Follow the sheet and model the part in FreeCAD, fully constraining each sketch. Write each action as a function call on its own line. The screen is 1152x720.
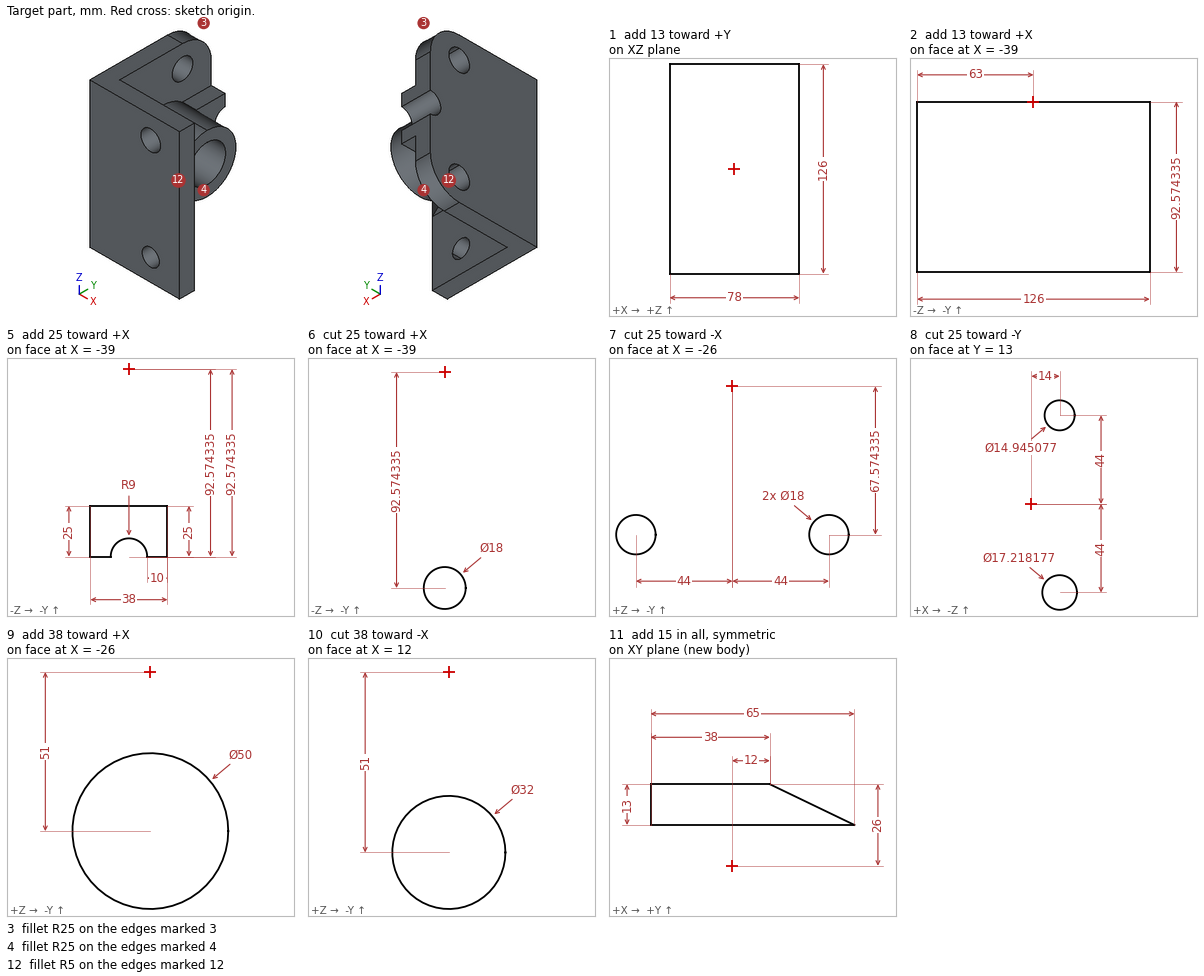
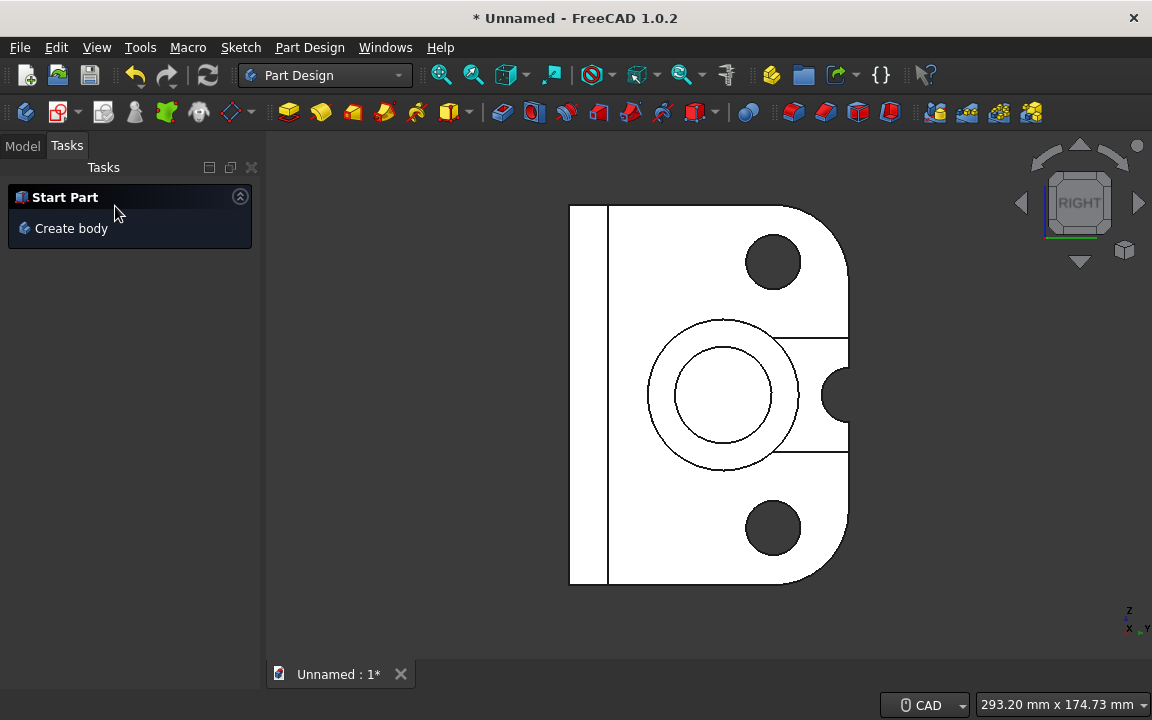
click(26, 112)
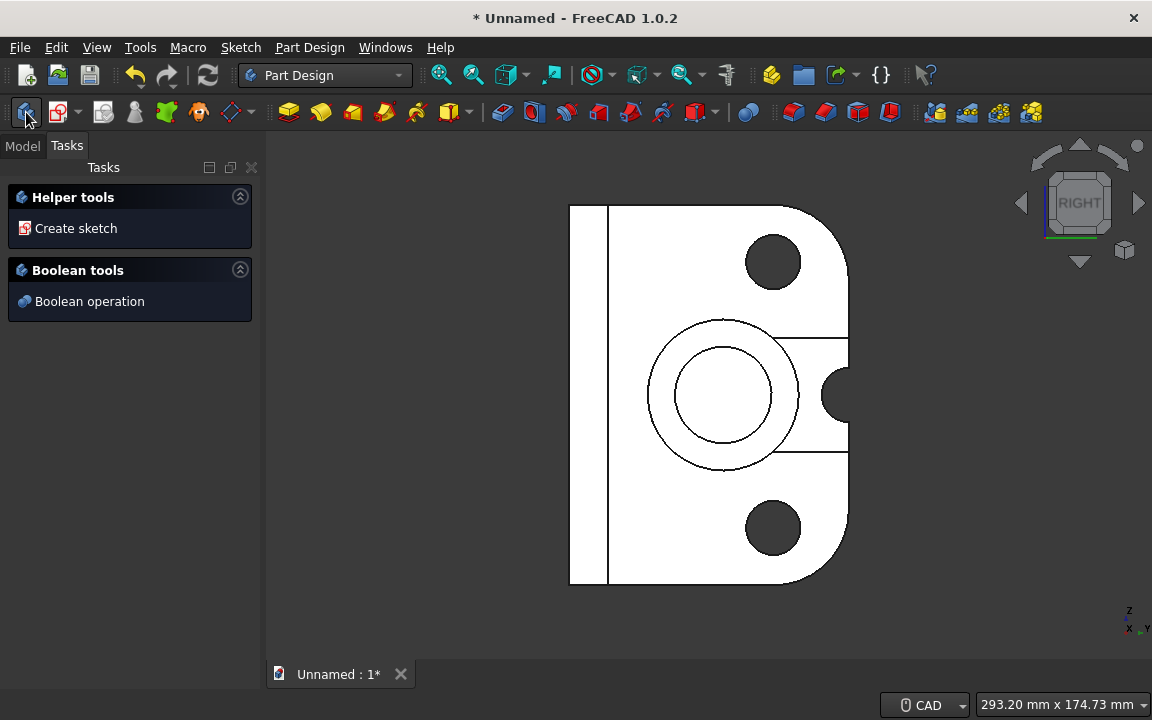
click(306, 619)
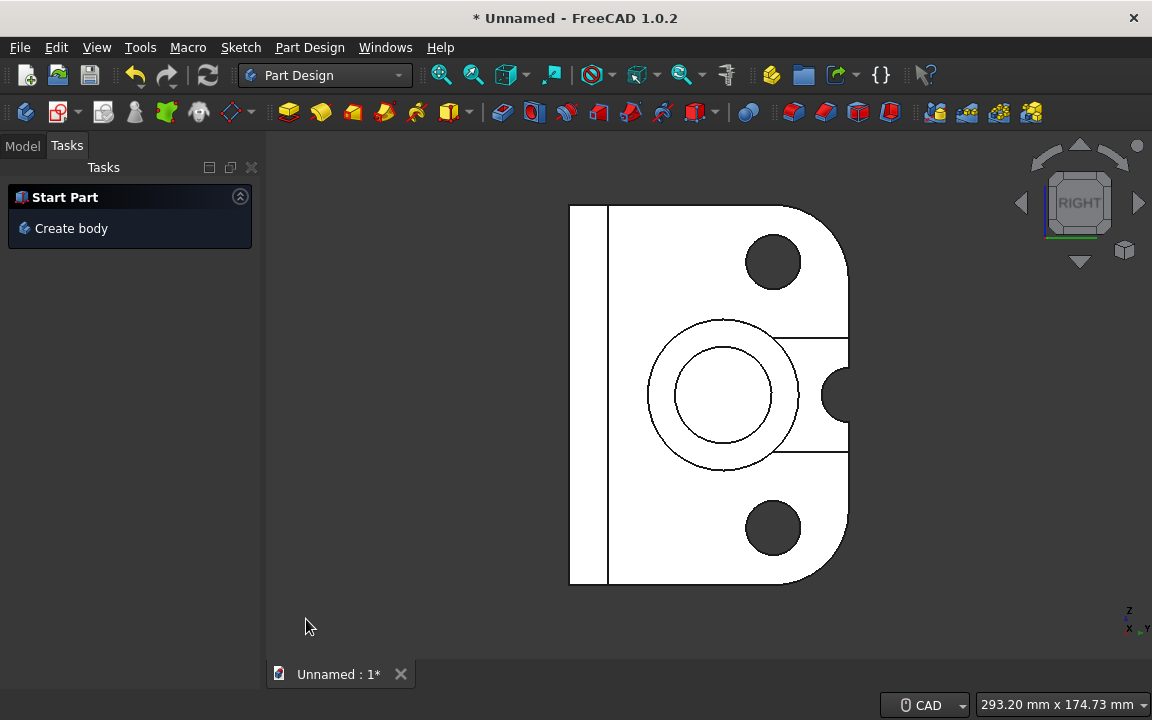
click(58, 112)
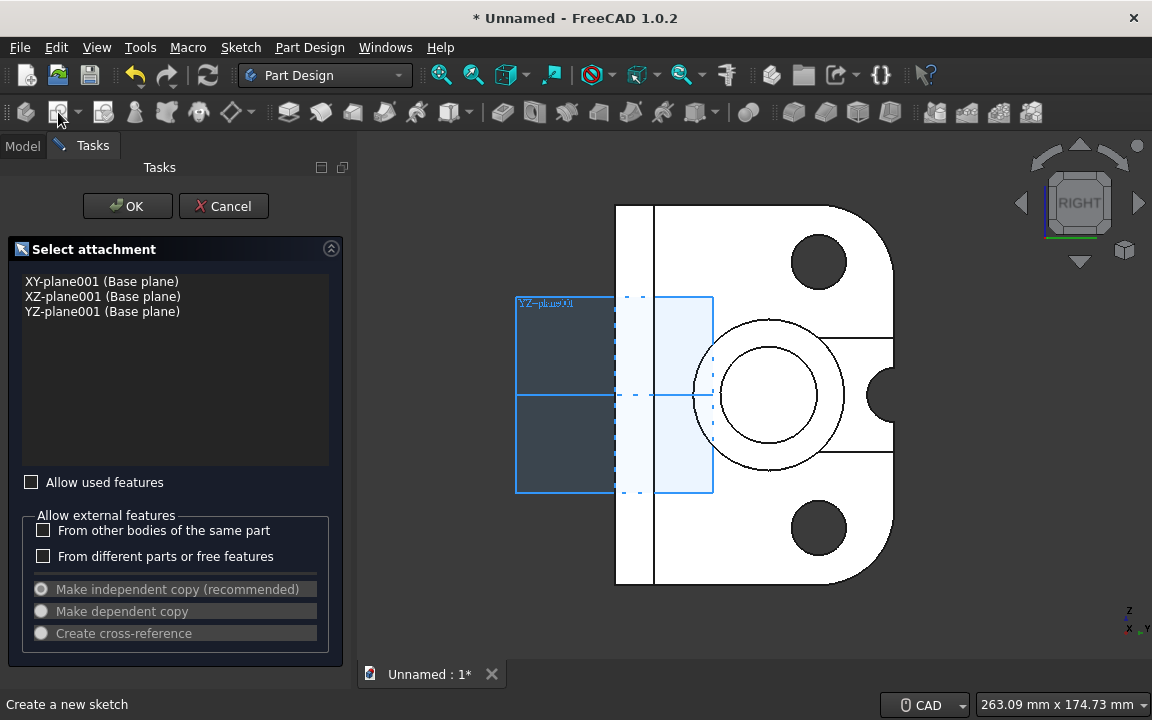
click(82, 282)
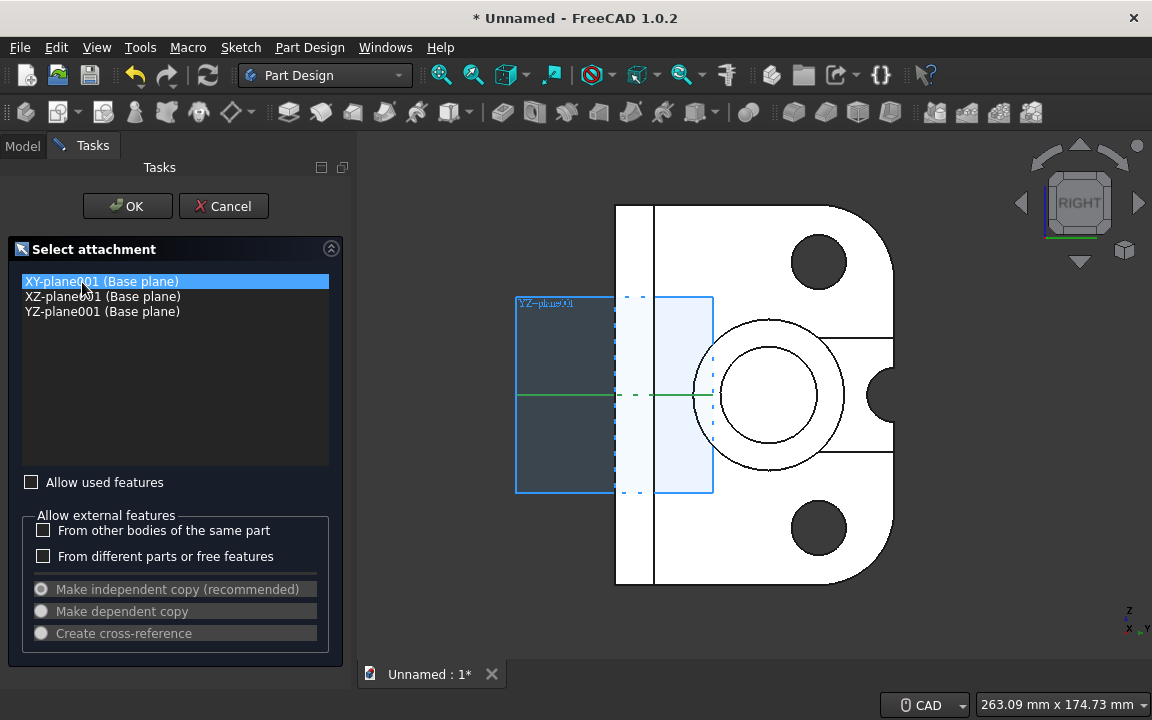
click(128, 206)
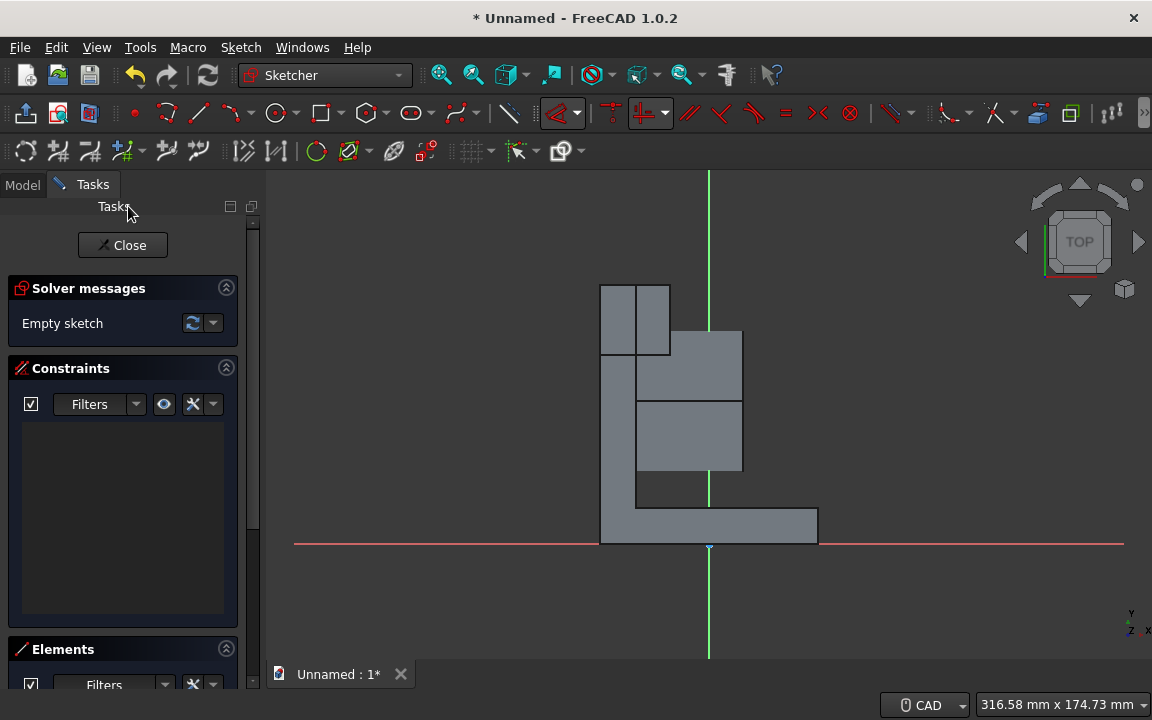
scroll(778, 562, up, 5)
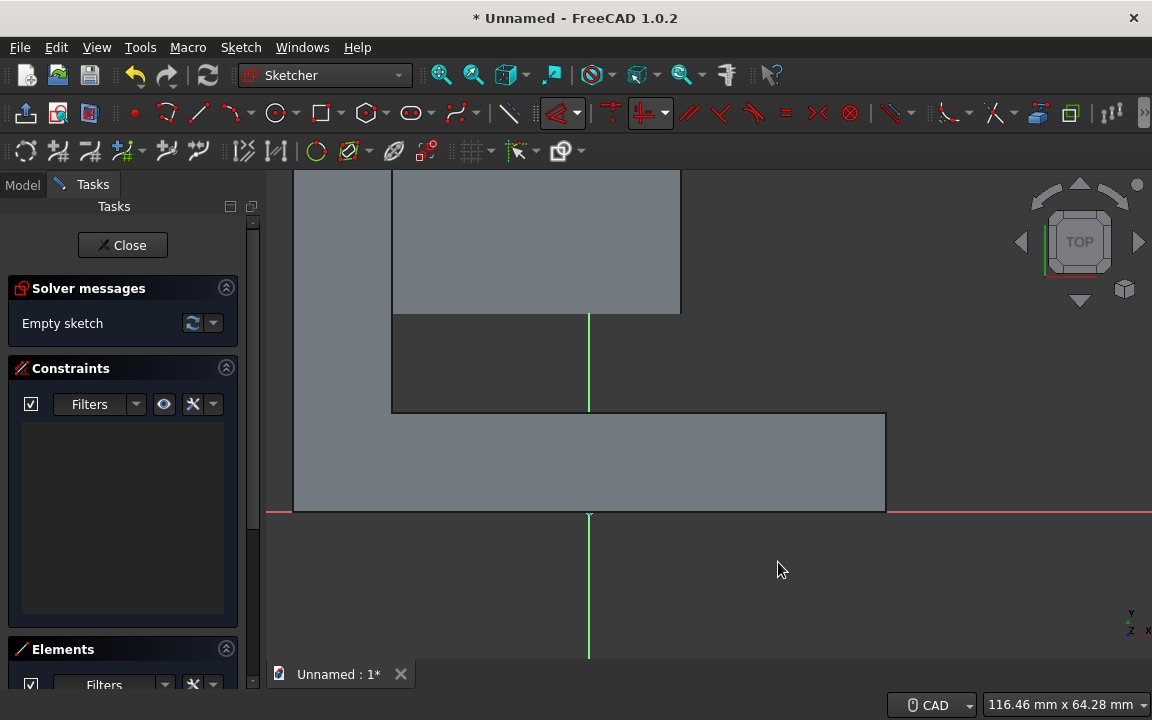
click(168, 114)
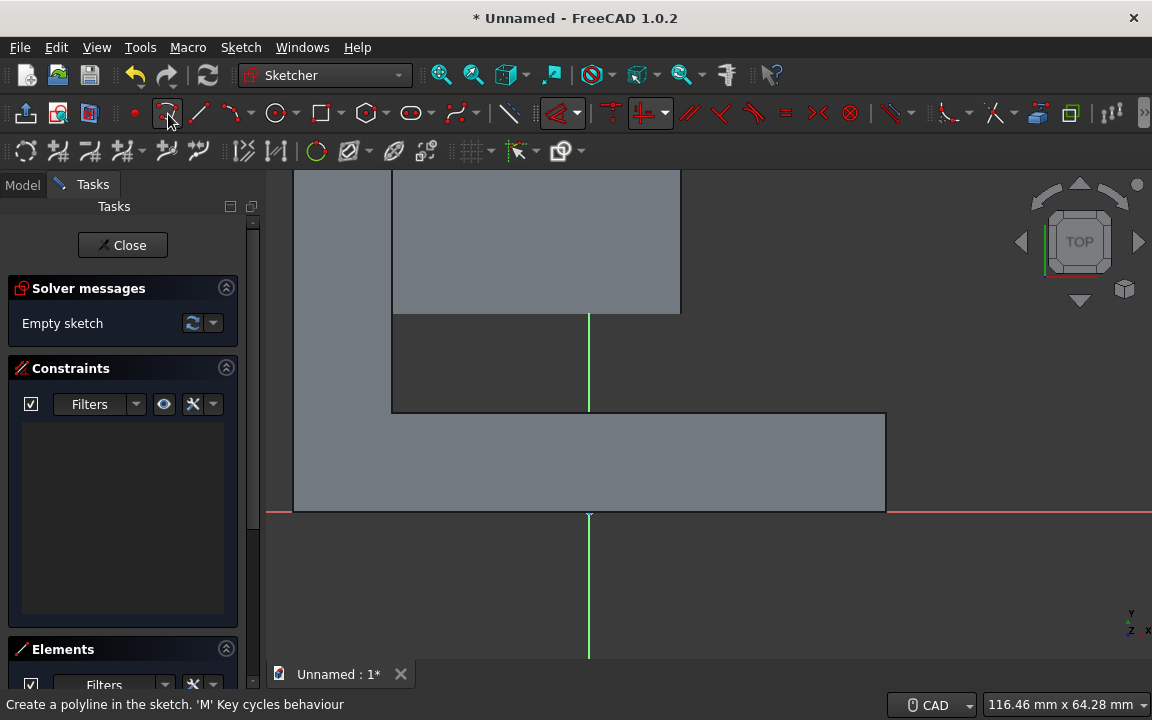
click(681, 314)
click(392, 314)
click(392, 413)
click(886, 413)
click(681, 315)
key(Escape)
key(Escape)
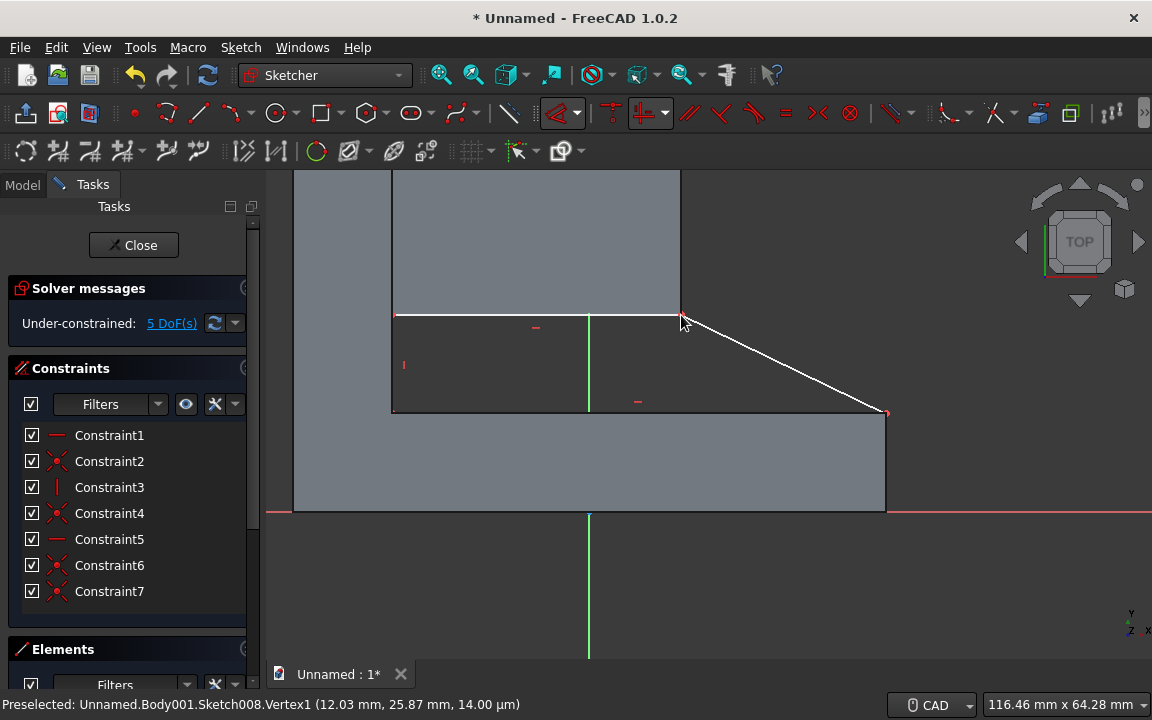
click(479, 315)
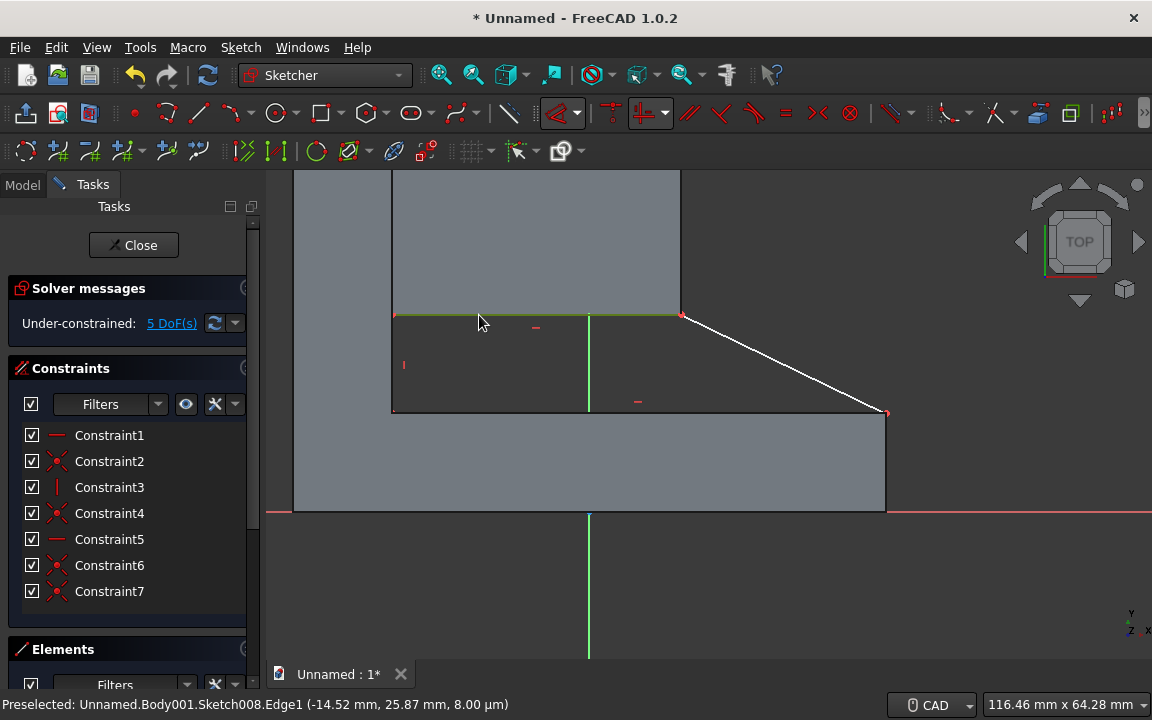
key(l)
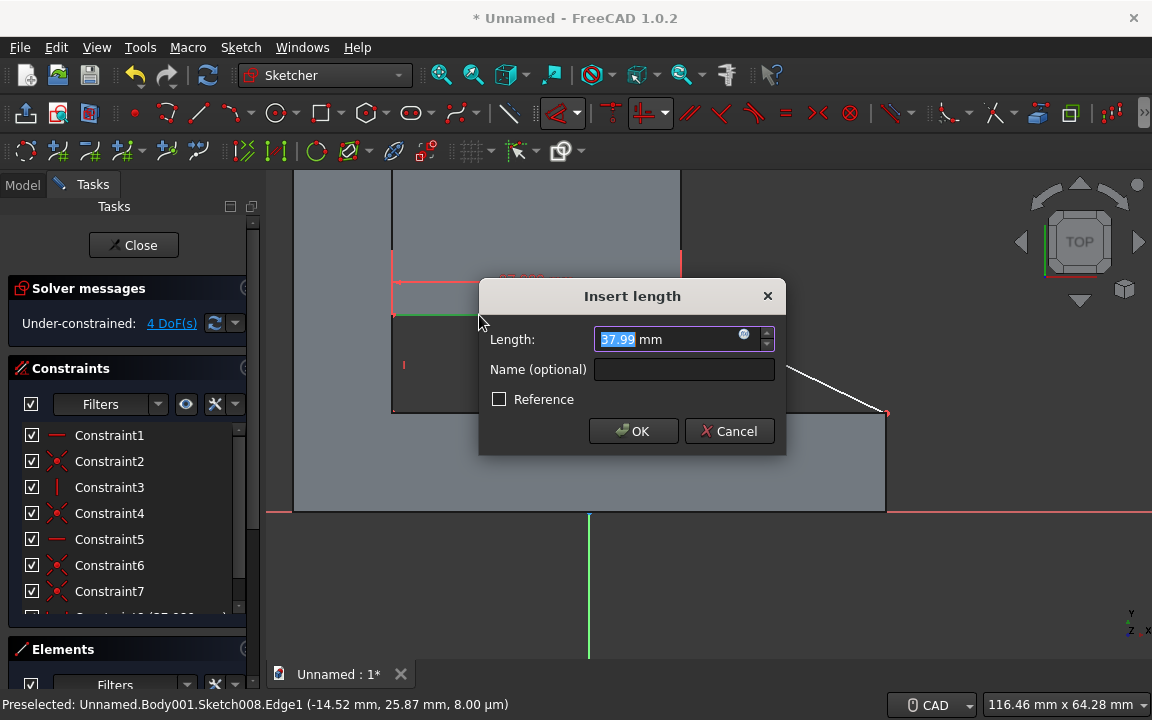
text(38)
key(Return)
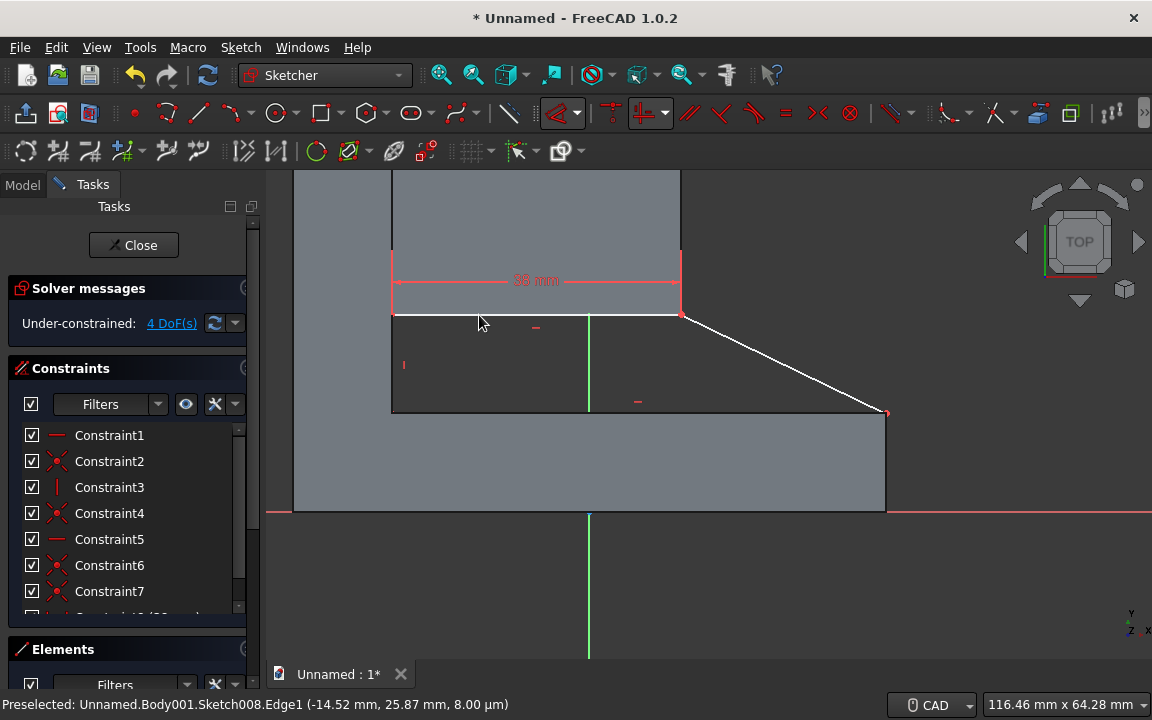
click(392, 345)